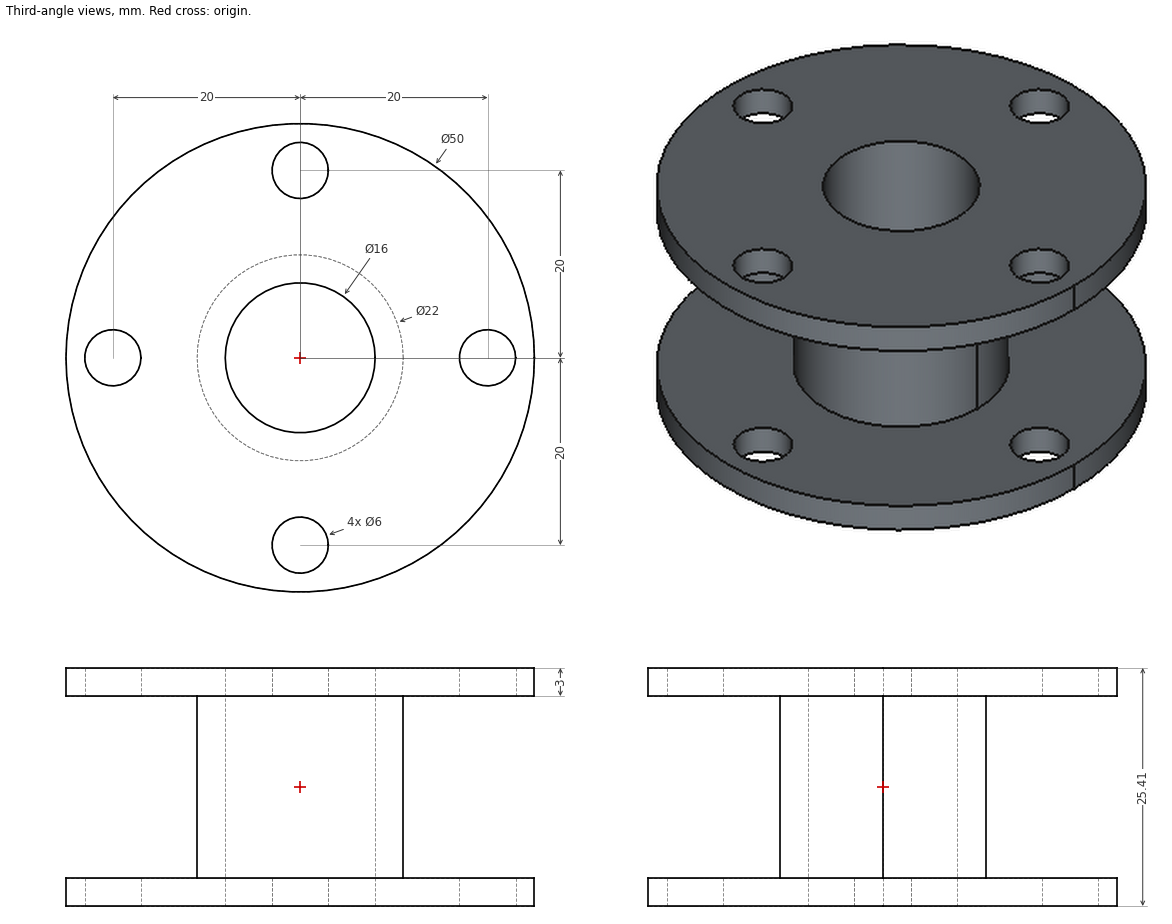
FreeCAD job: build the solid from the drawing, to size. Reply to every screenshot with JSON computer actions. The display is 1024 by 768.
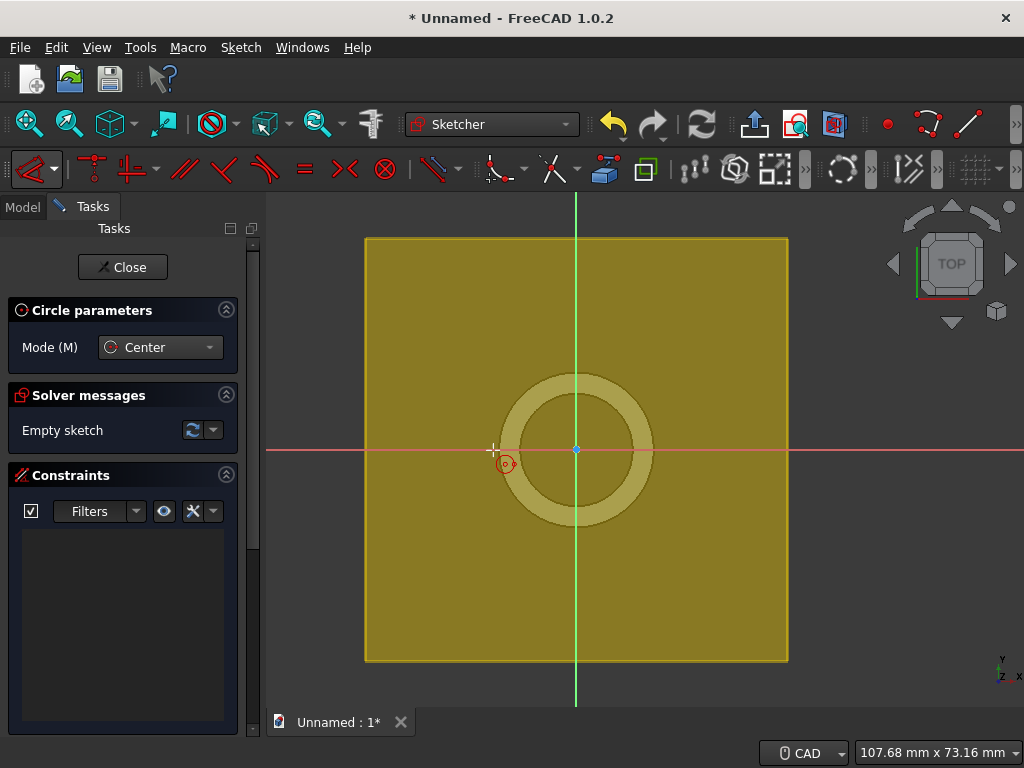
{"action": "left_click", "coordinate": [576, 450]}
{"action": "left_click", "coordinate": [701, 326]}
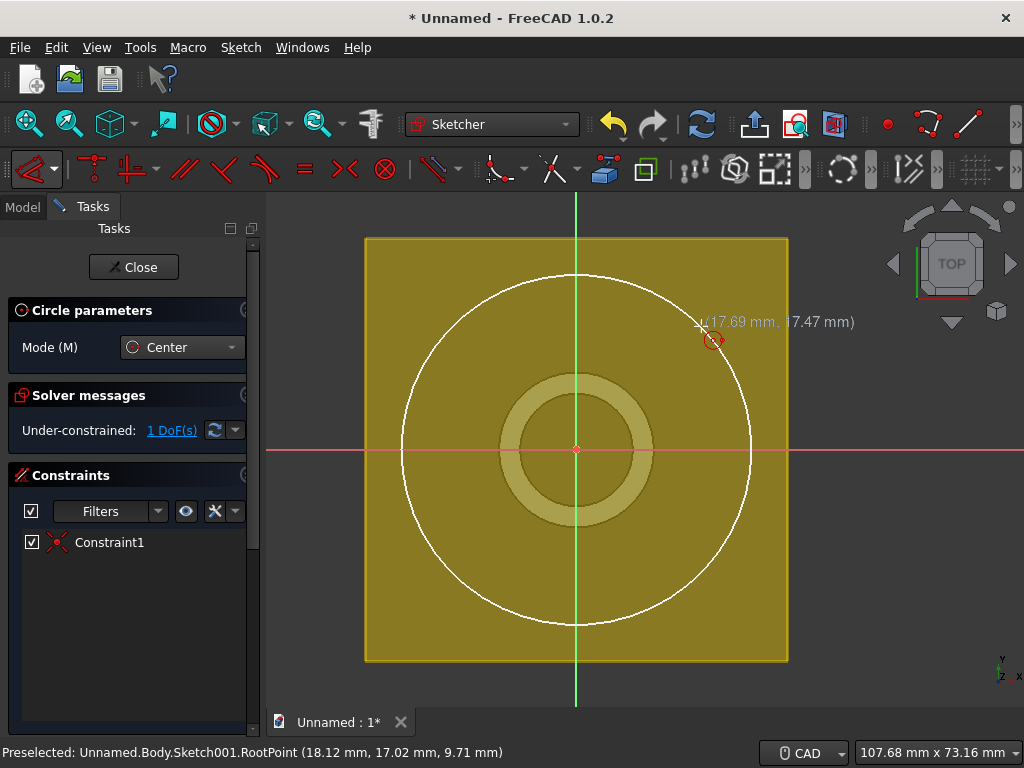
{"action": "left_click", "coordinate": [576, 591]}
{"action": "left_click", "coordinate": [591, 576]}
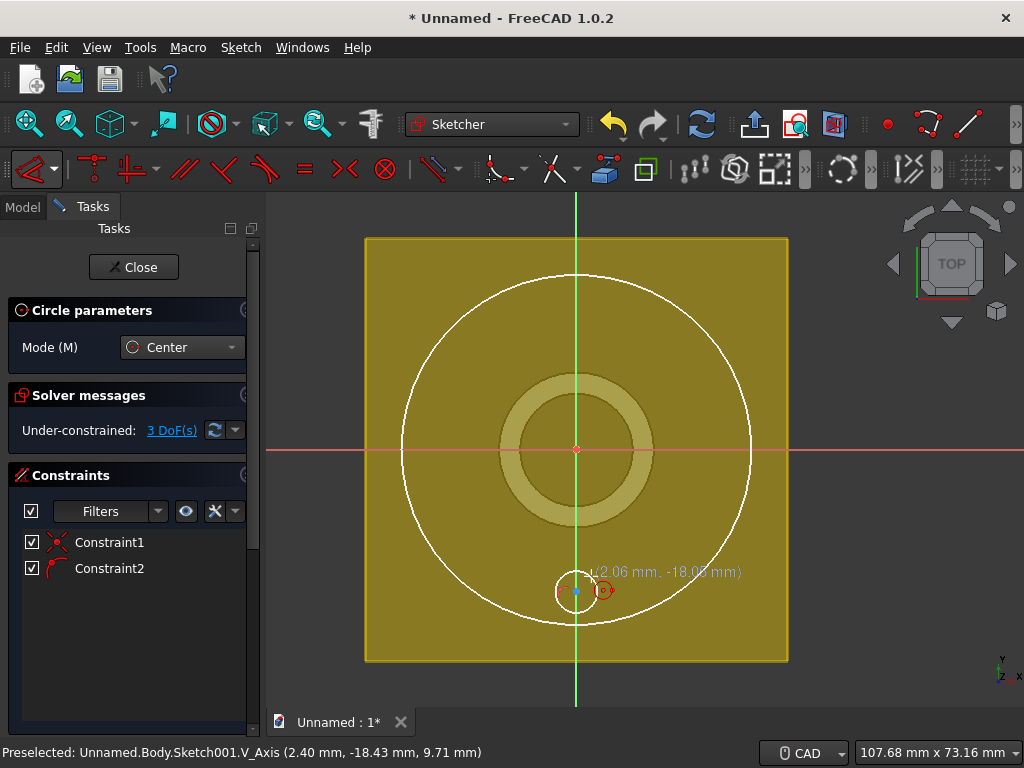
{"action": "left_click", "coordinate": [436, 450]}
{"action": "left_click", "coordinate": [451, 435]}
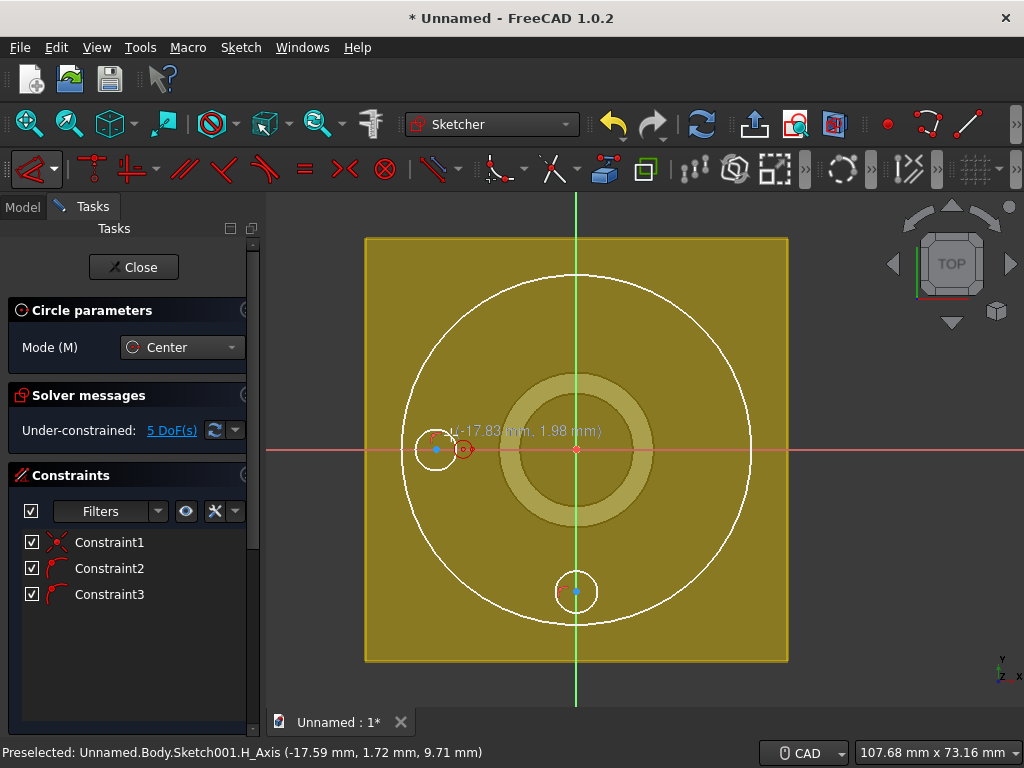
{"action": "left_click", "coordinate": [576, 450]}
{"action": "left_click", "coordinate": [616, 410]}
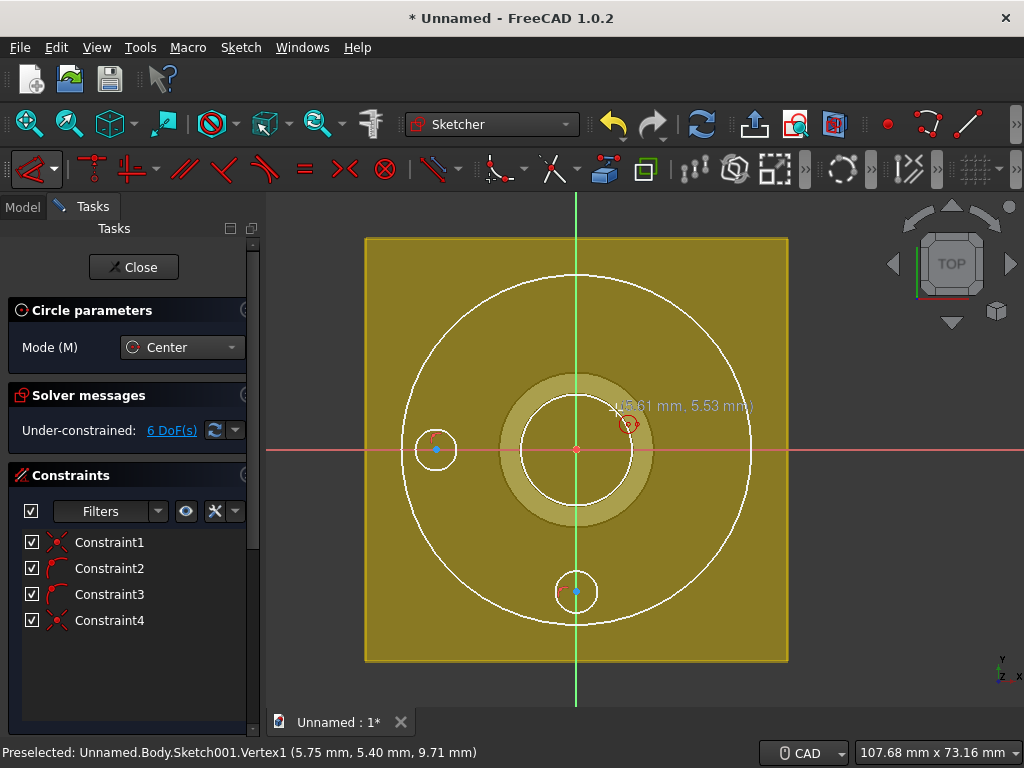
{"action": "left_click", "coordinate": [717, 450]}
{"action": "left_click", "coordinate": [732, 435]}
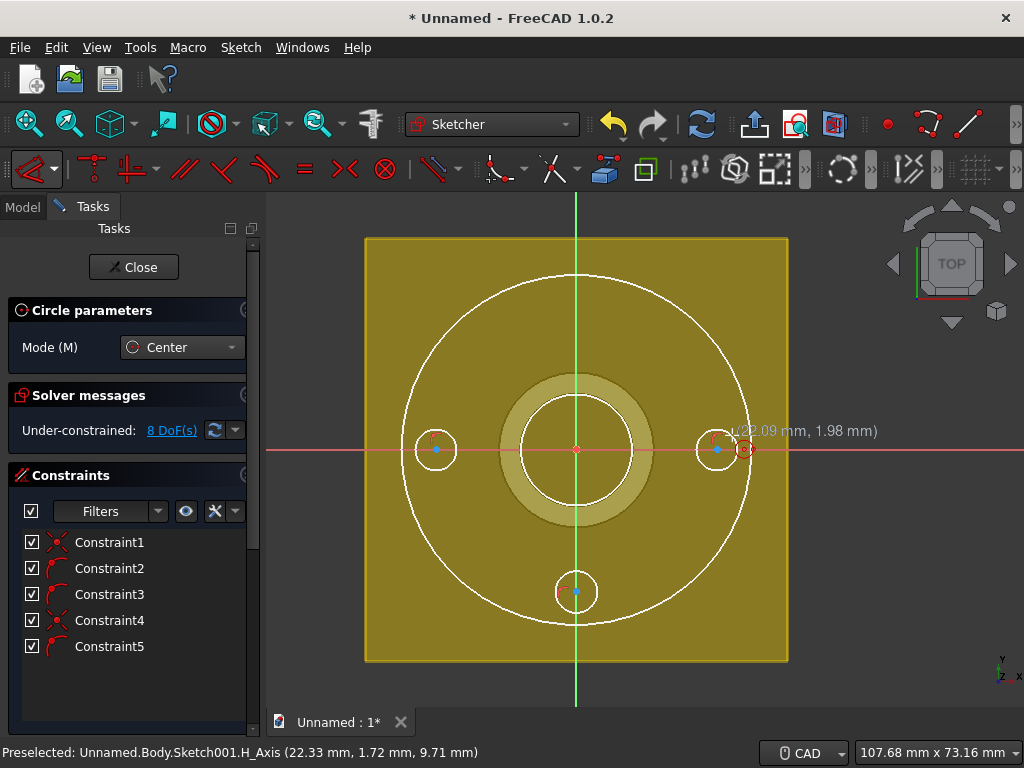
{"action": "left_click", "coordinate": [576, 309]}
{"action": "left_click", "coordinate": [591, 294]}
{"action": "key", "text": "Escape"}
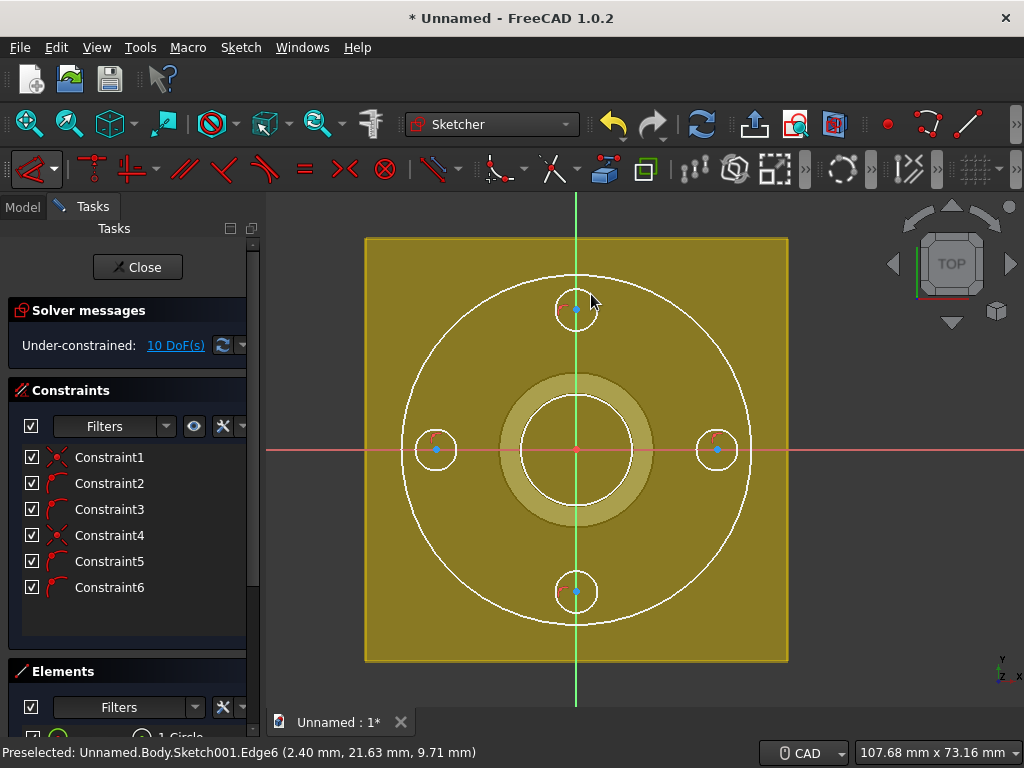
{"action": "left_click", "coordinate": [591, 577]}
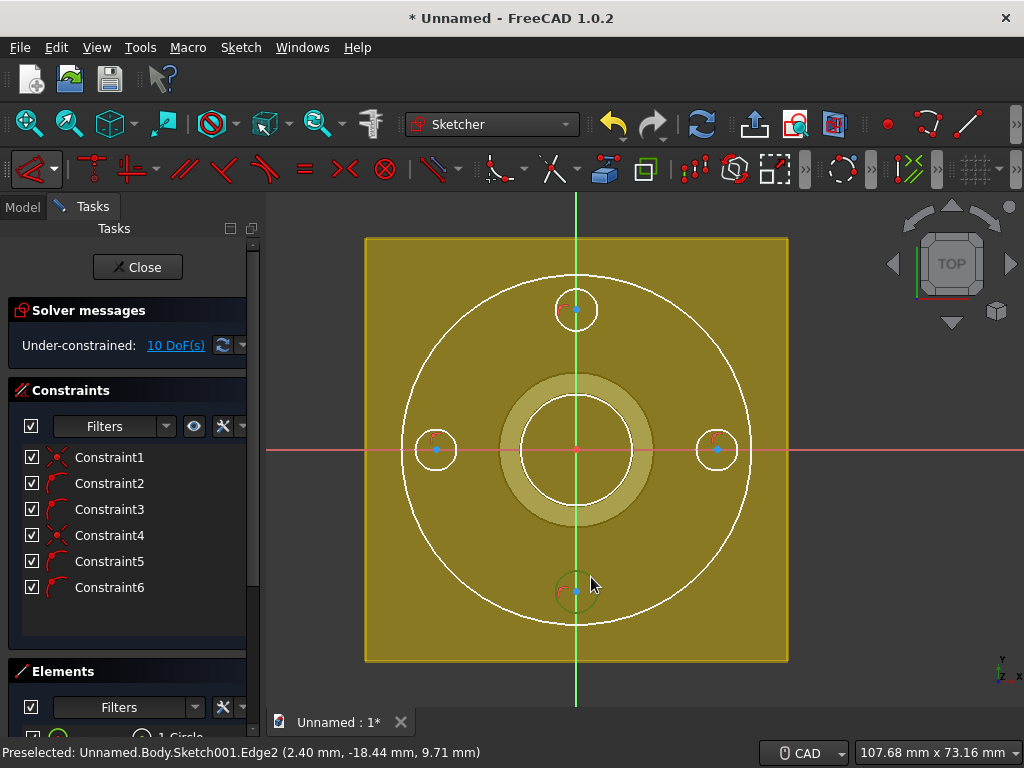
{"action": "left_click", "coordinate": [450, 435]}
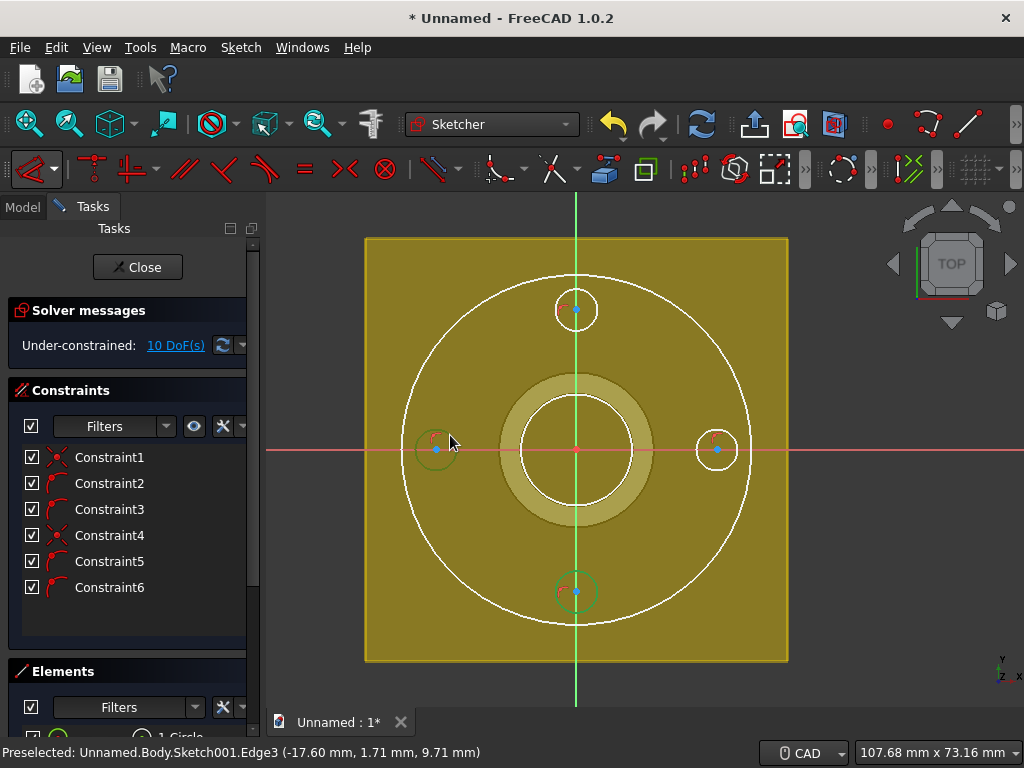
{"action": "left_click", "coordinate": [731, 435]}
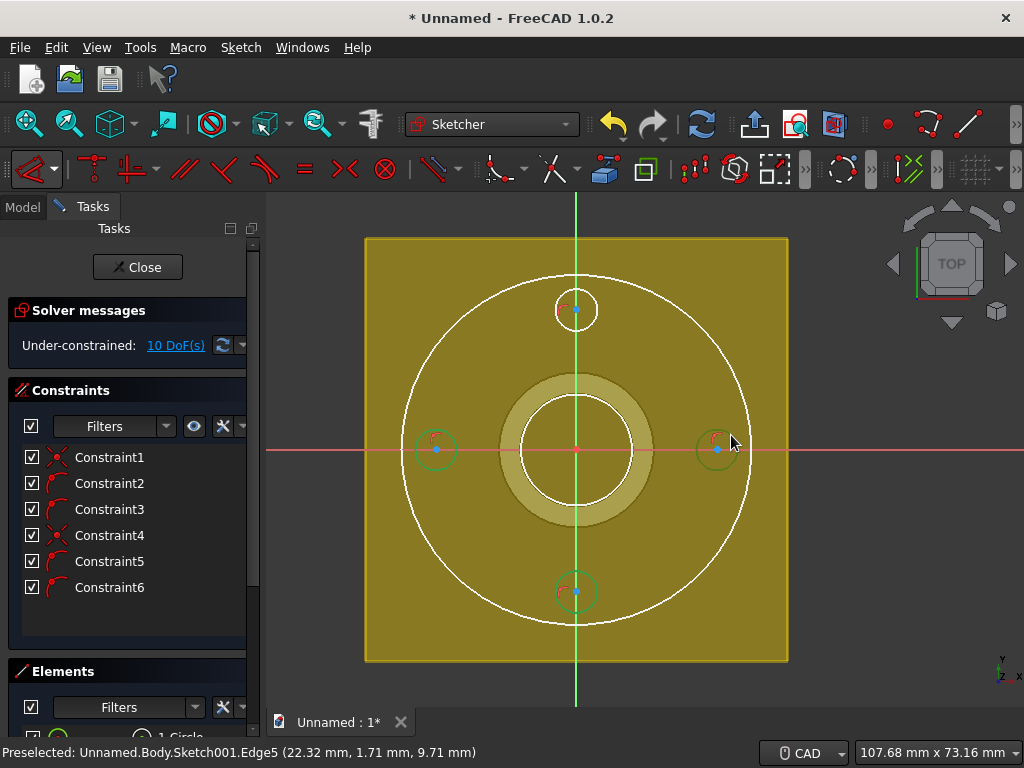
{"action": "left_click", "coordinate": [591, 295]}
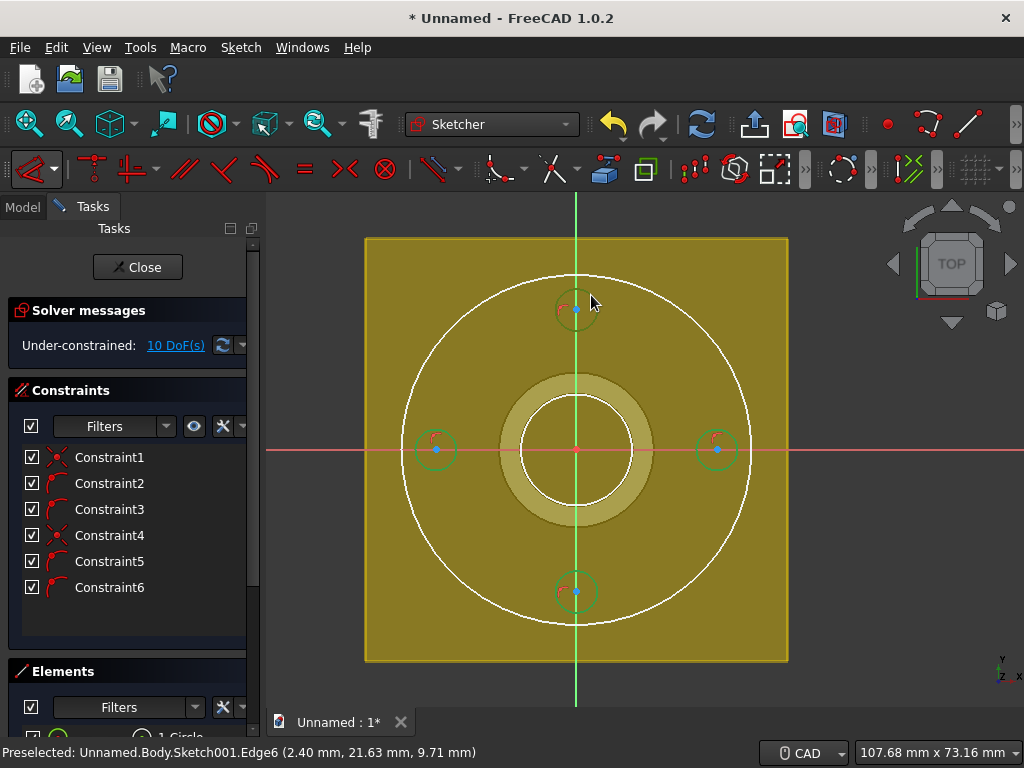
{"action": "left_click", "coordinate": [306, 170]}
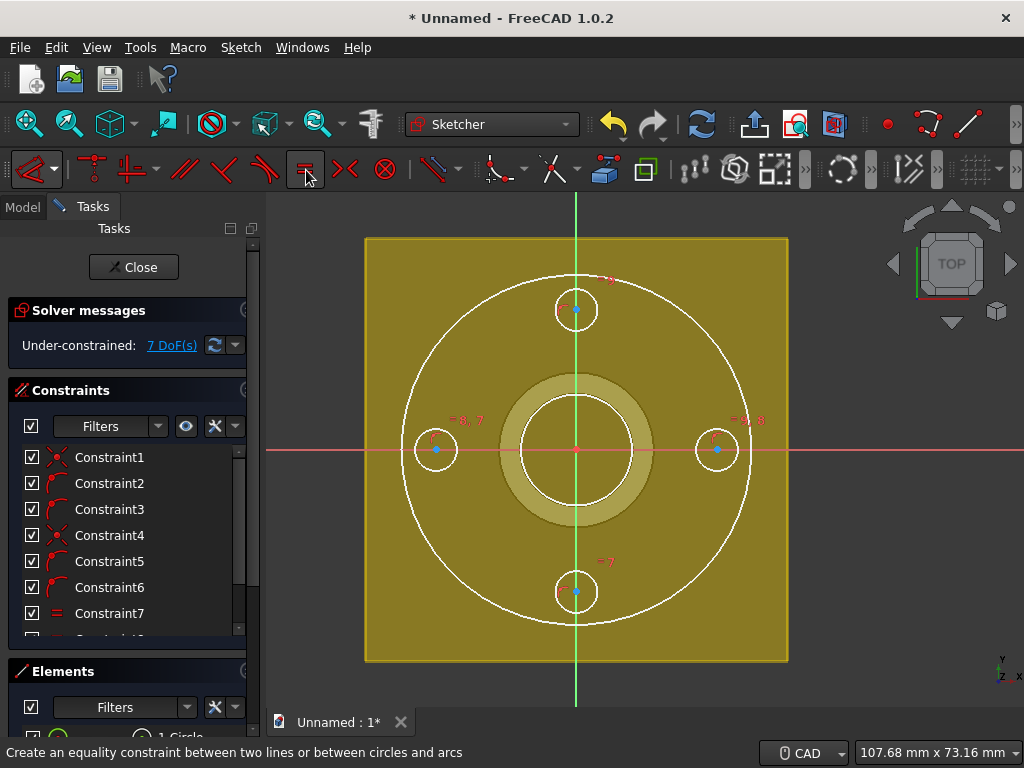
{"action": "left_click", "coordinate": [700, 326]}